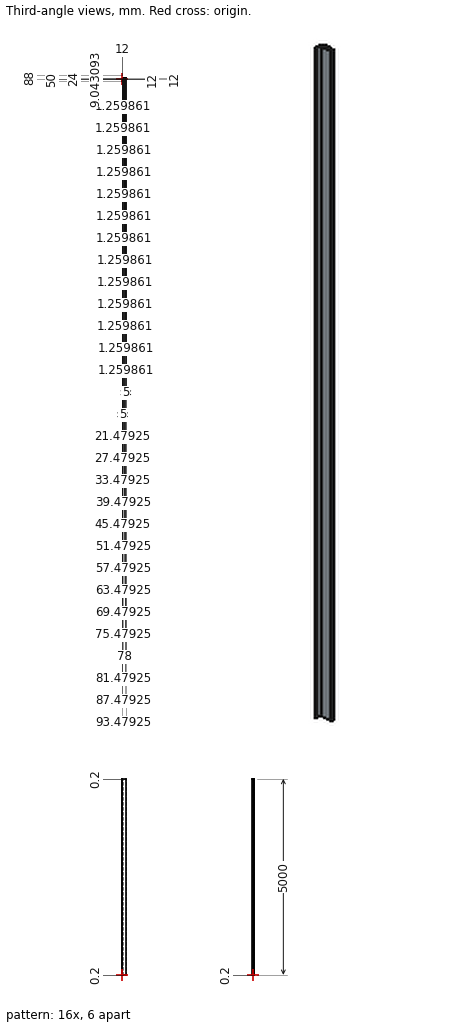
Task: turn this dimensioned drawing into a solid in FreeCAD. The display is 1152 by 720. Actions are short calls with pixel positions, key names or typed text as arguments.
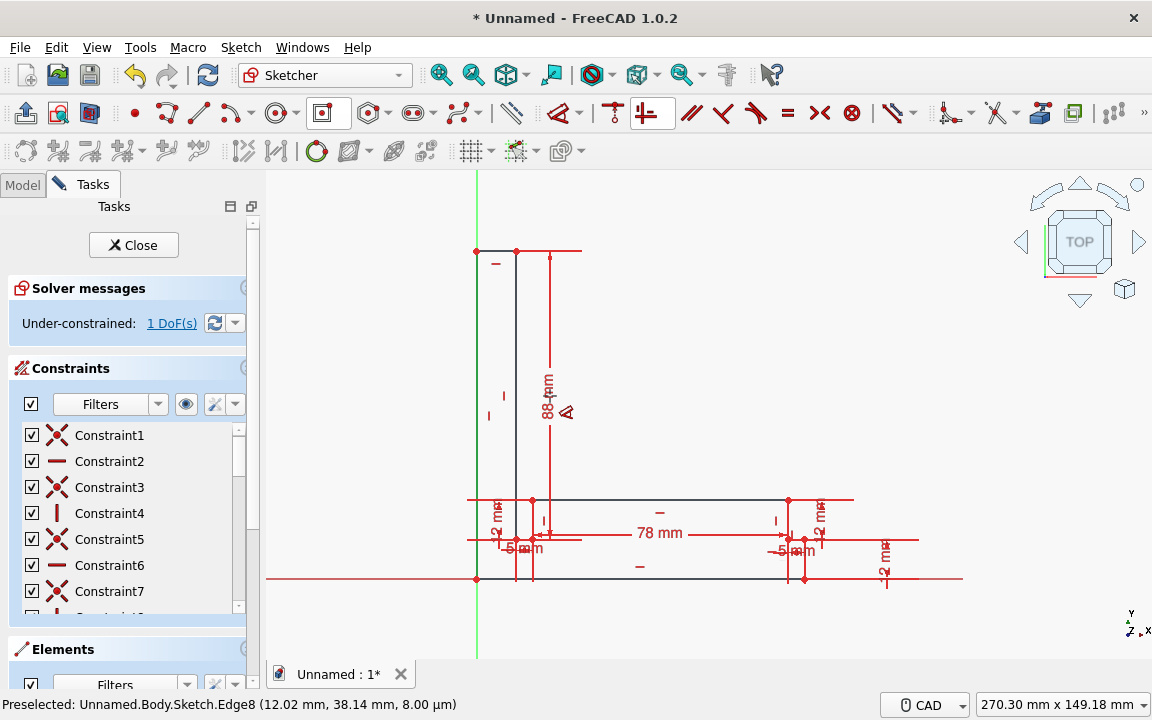
click(504, 251)
click(497, 217)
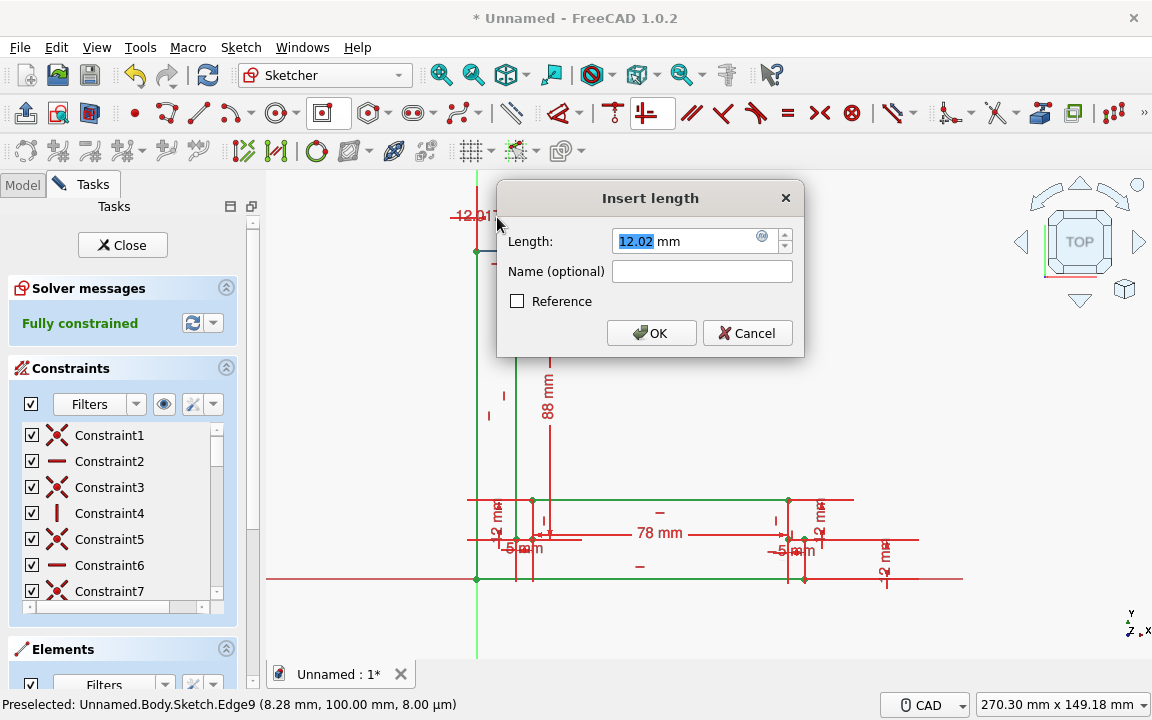
text(12)
key(Return)
key(Escape)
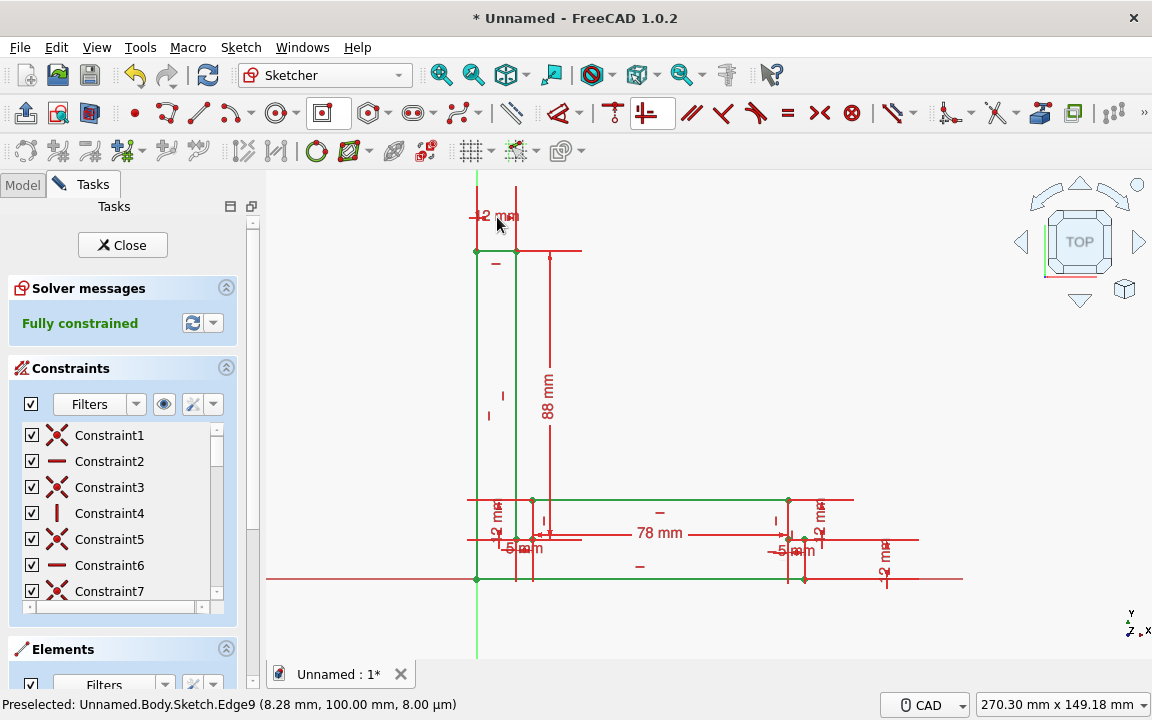
click(123, 245)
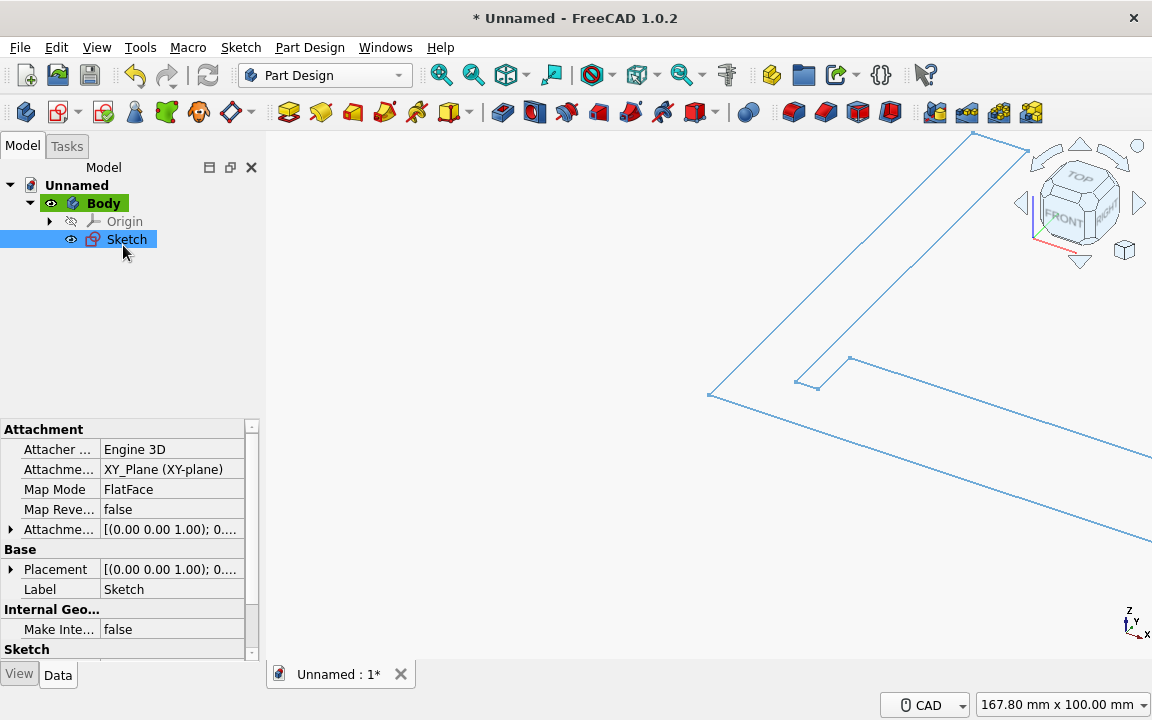
click(290, 112)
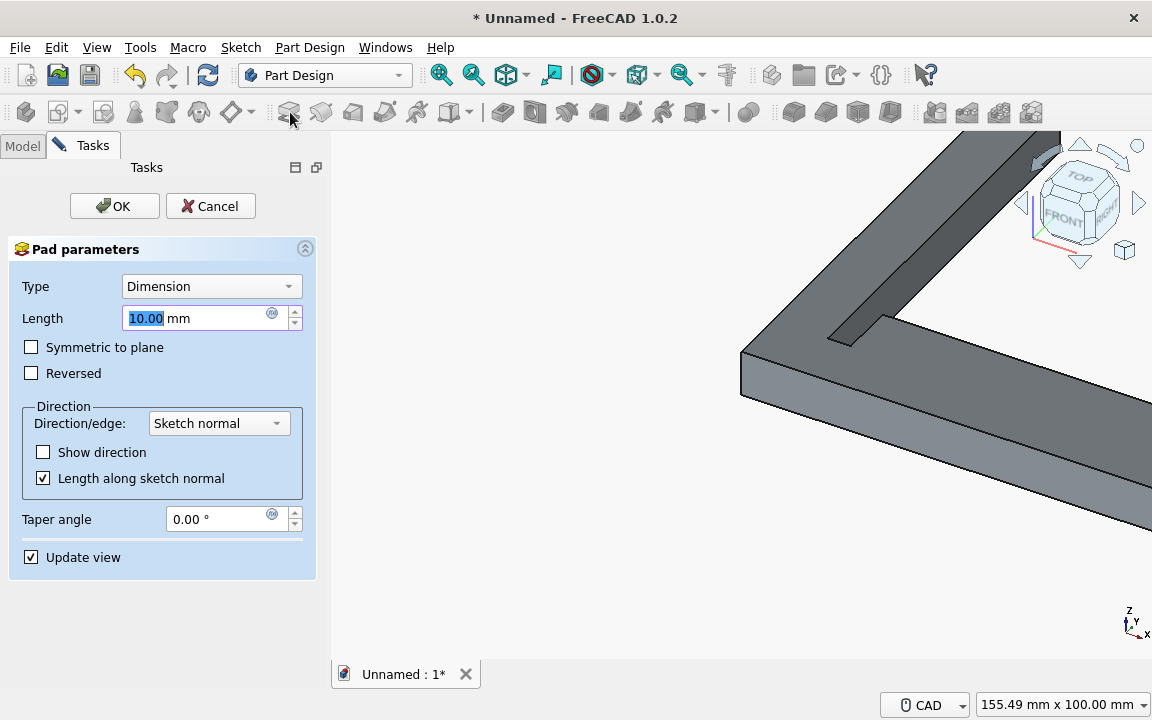
text(5000)
key(Tab)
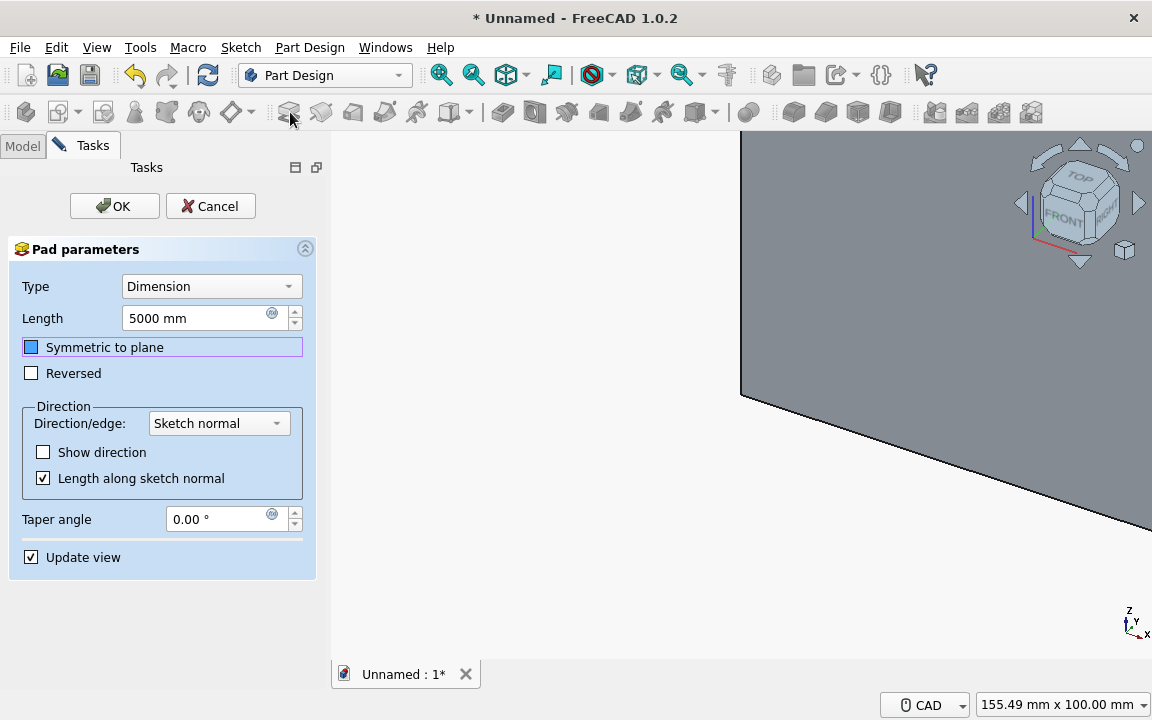
click(115, 206)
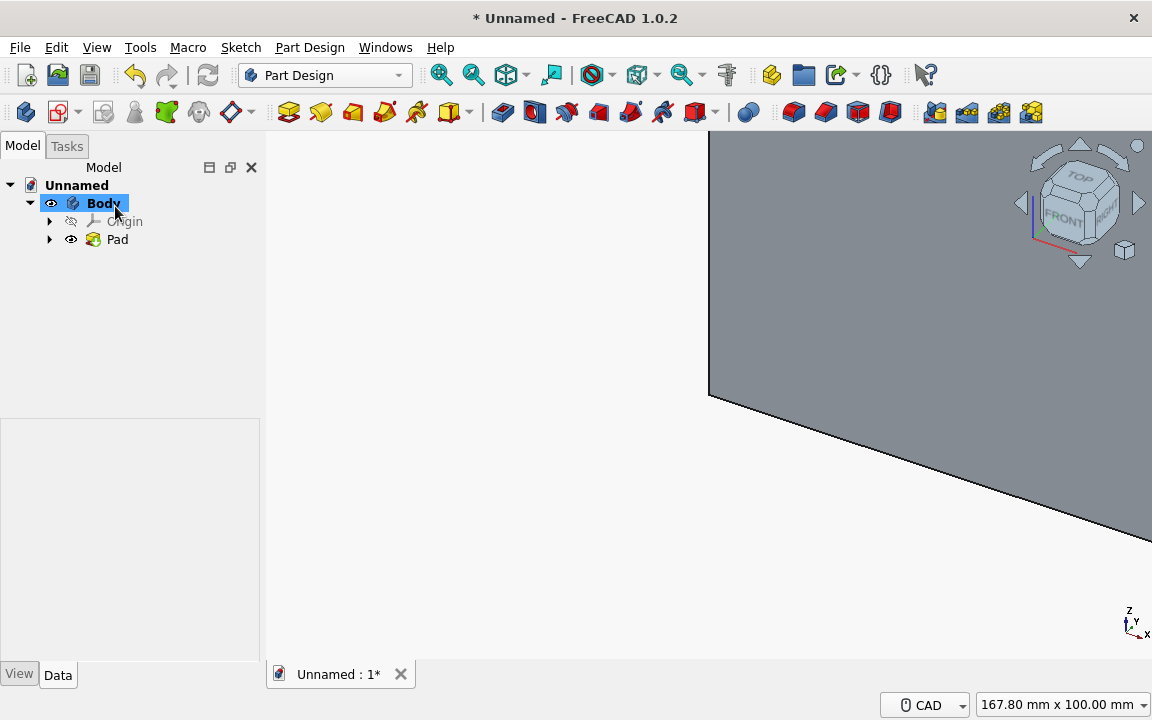
key(v)
key(f)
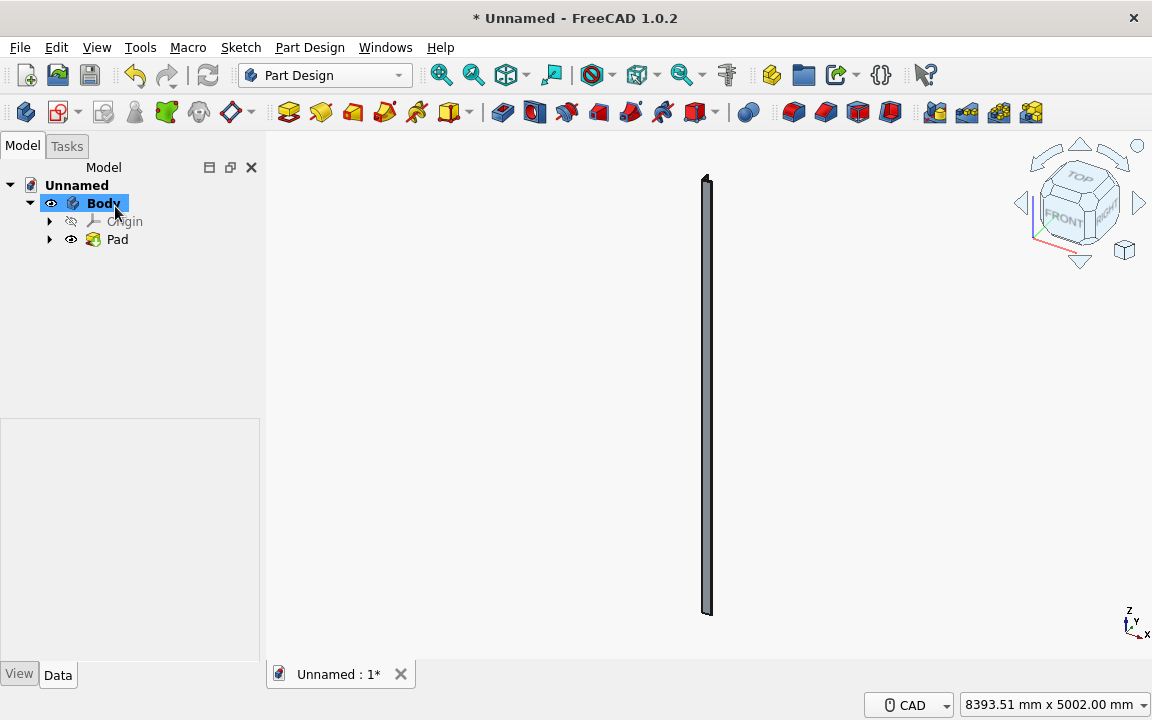
scroll(709, 181, up, 14)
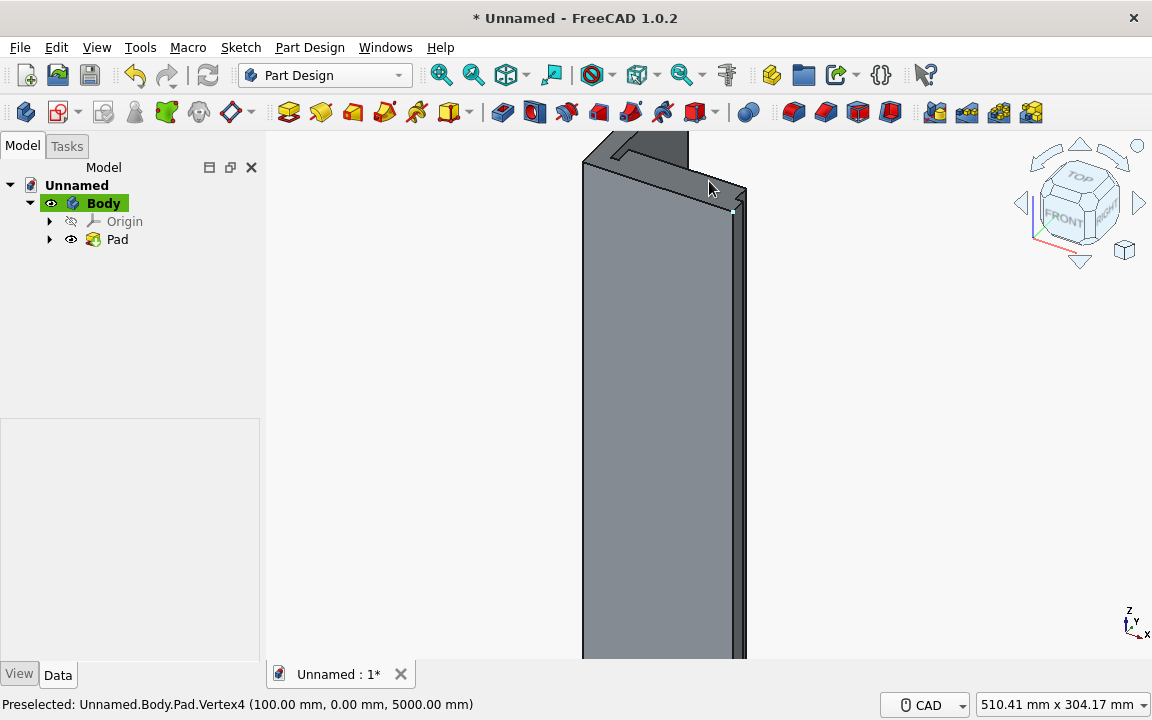
click(442, 76)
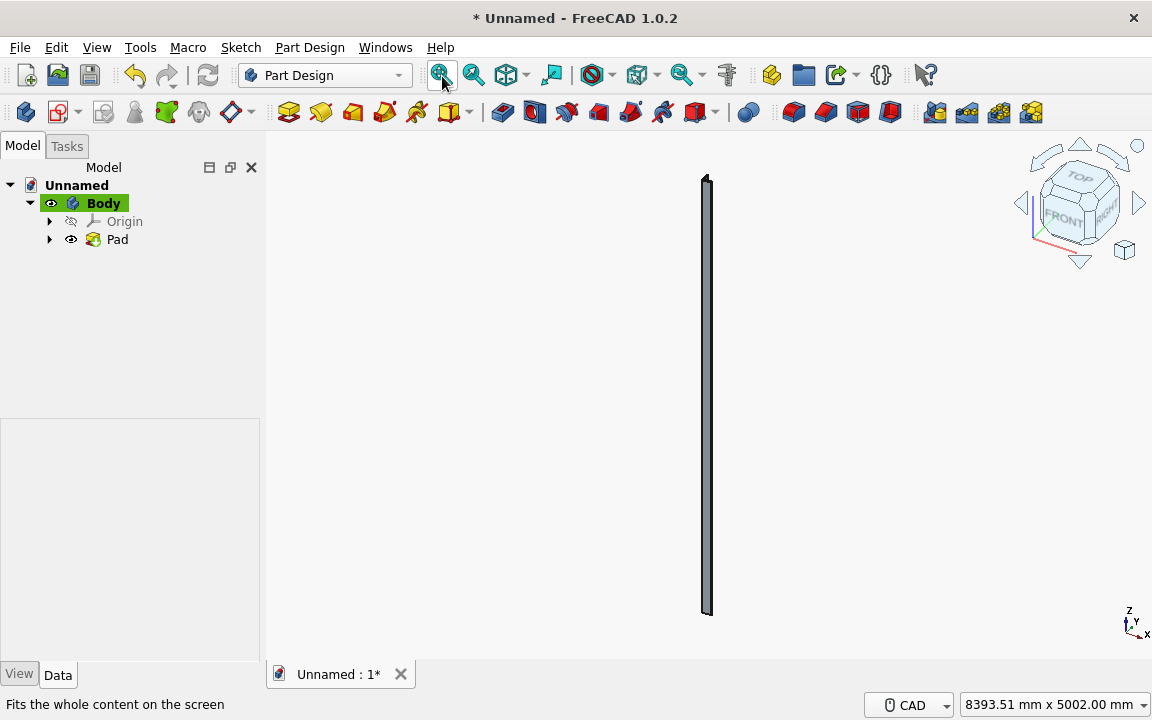
key(0)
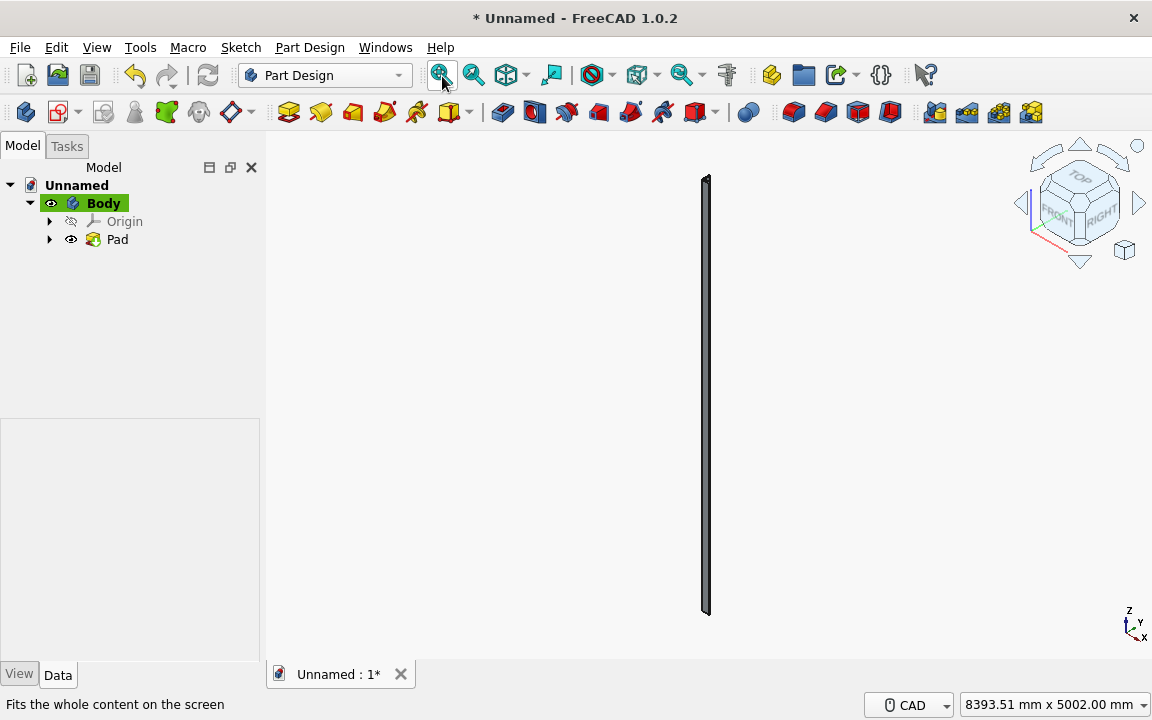
scroll(708, 182, up, 14)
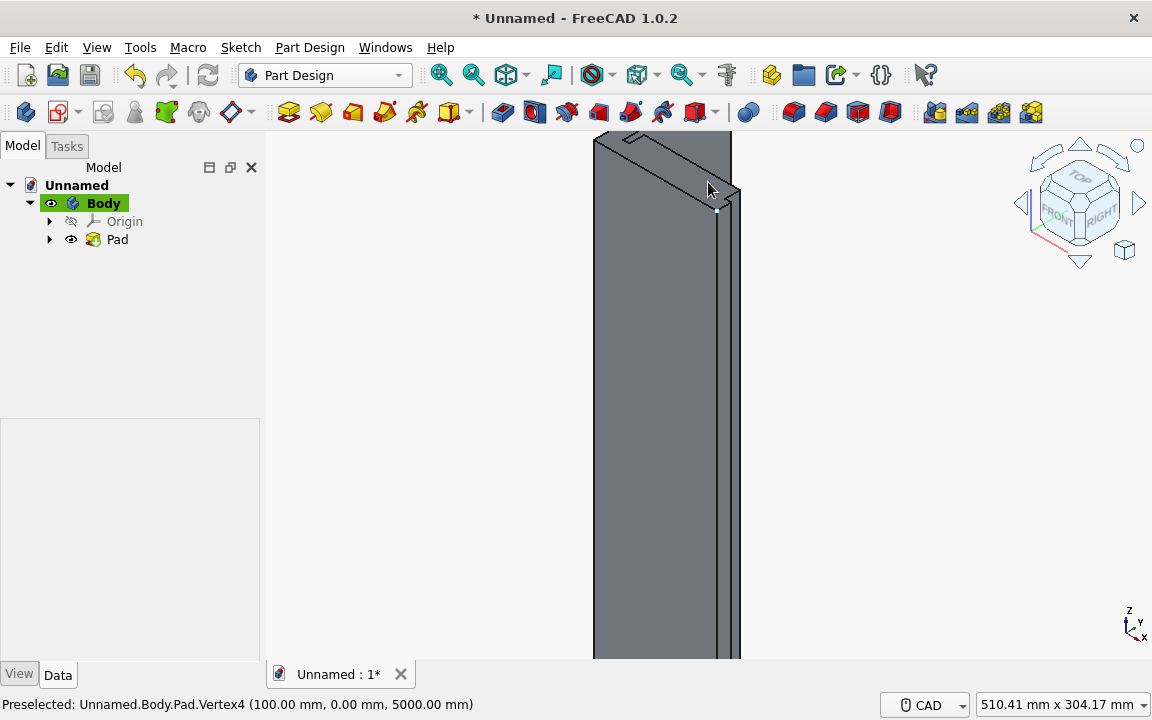
click(682, 179)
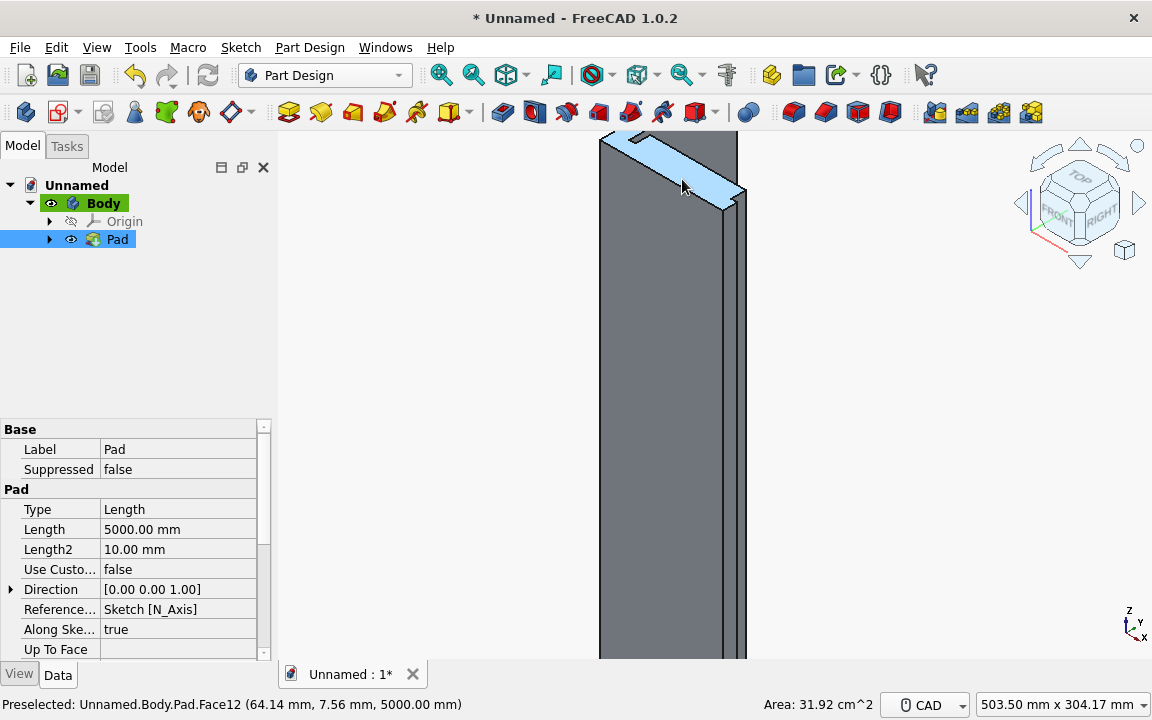
click(58, 112)